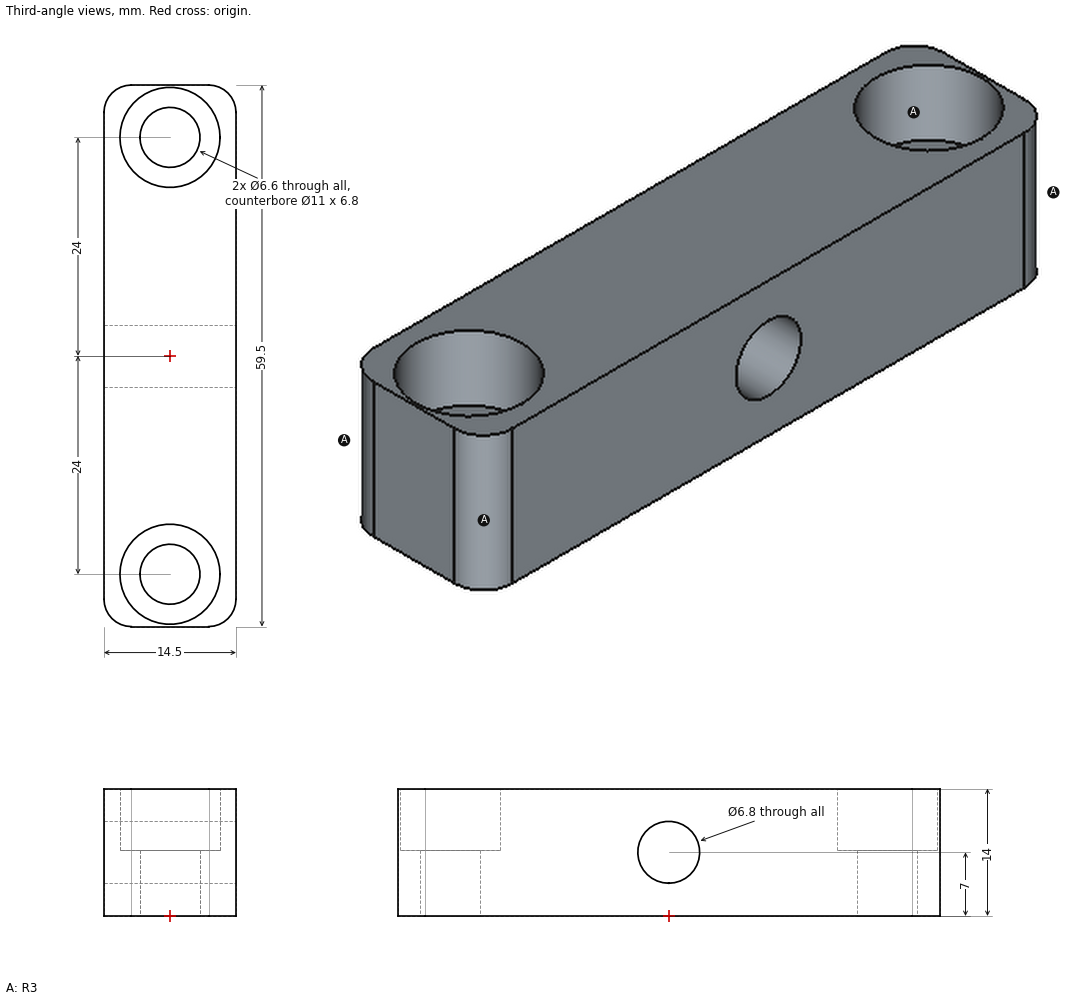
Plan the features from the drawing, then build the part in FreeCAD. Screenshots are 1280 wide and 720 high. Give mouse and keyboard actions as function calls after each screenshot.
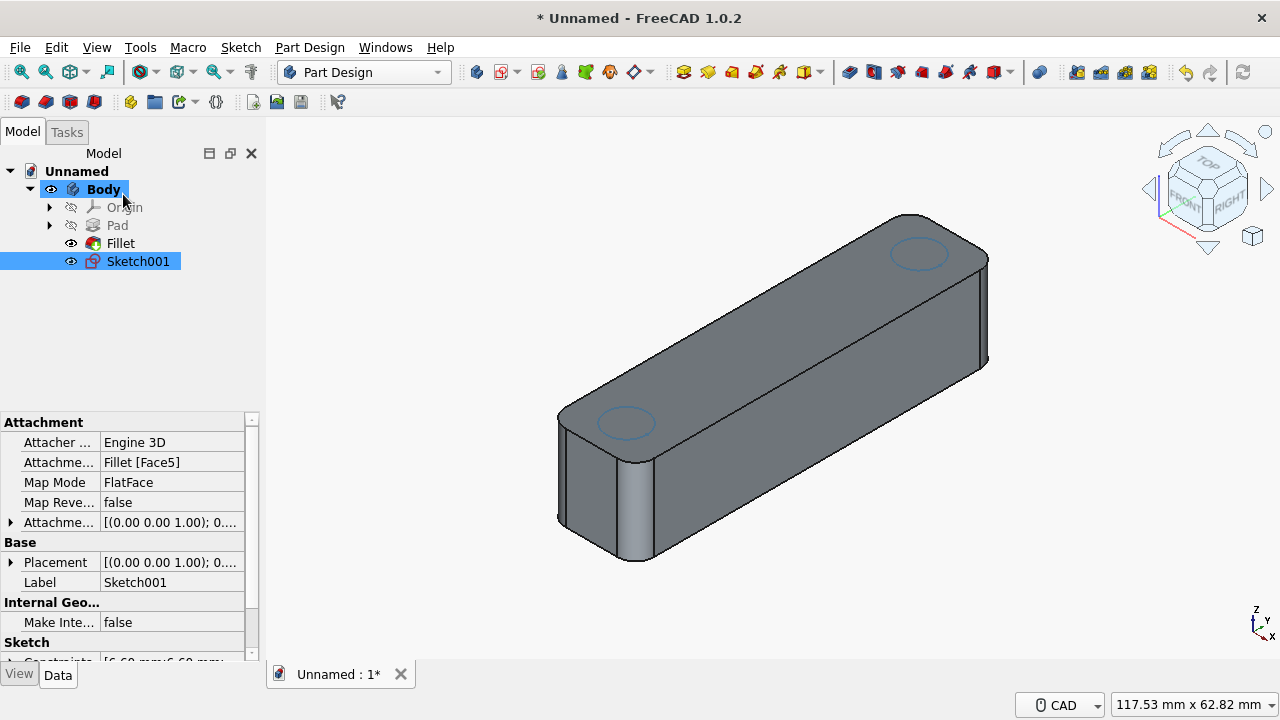
click(874, 72)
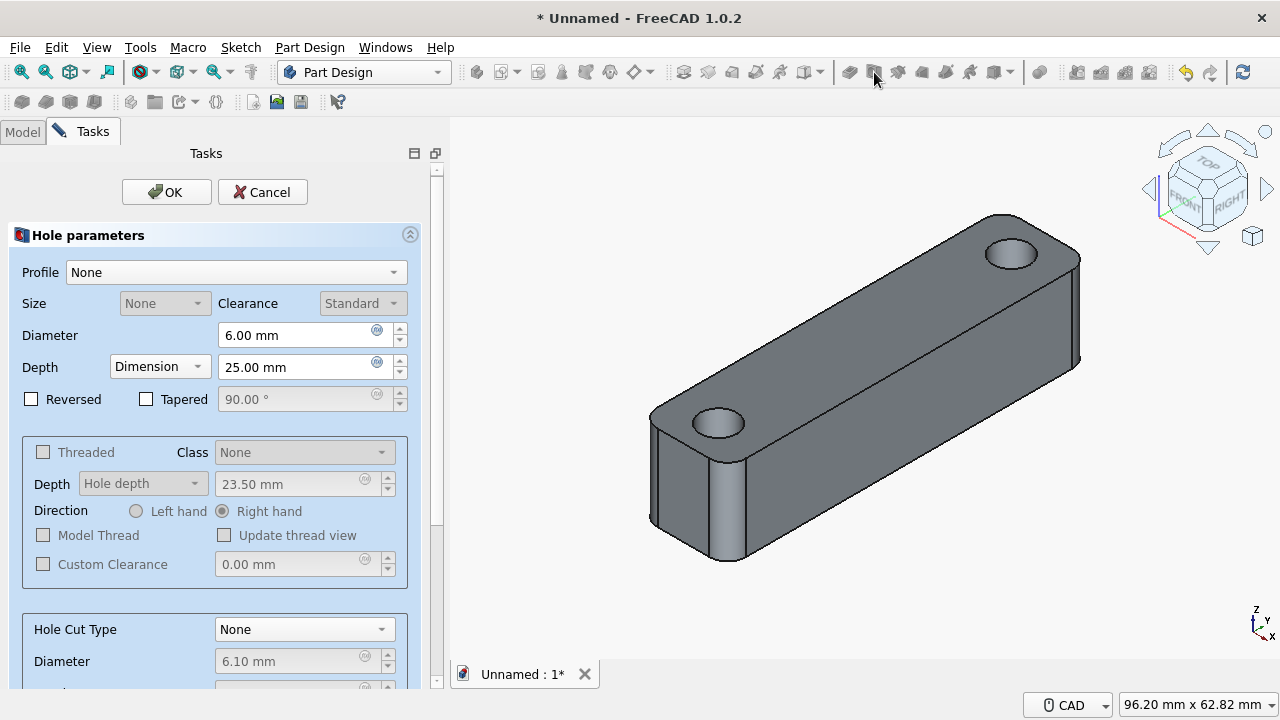
triple_click(305, 335)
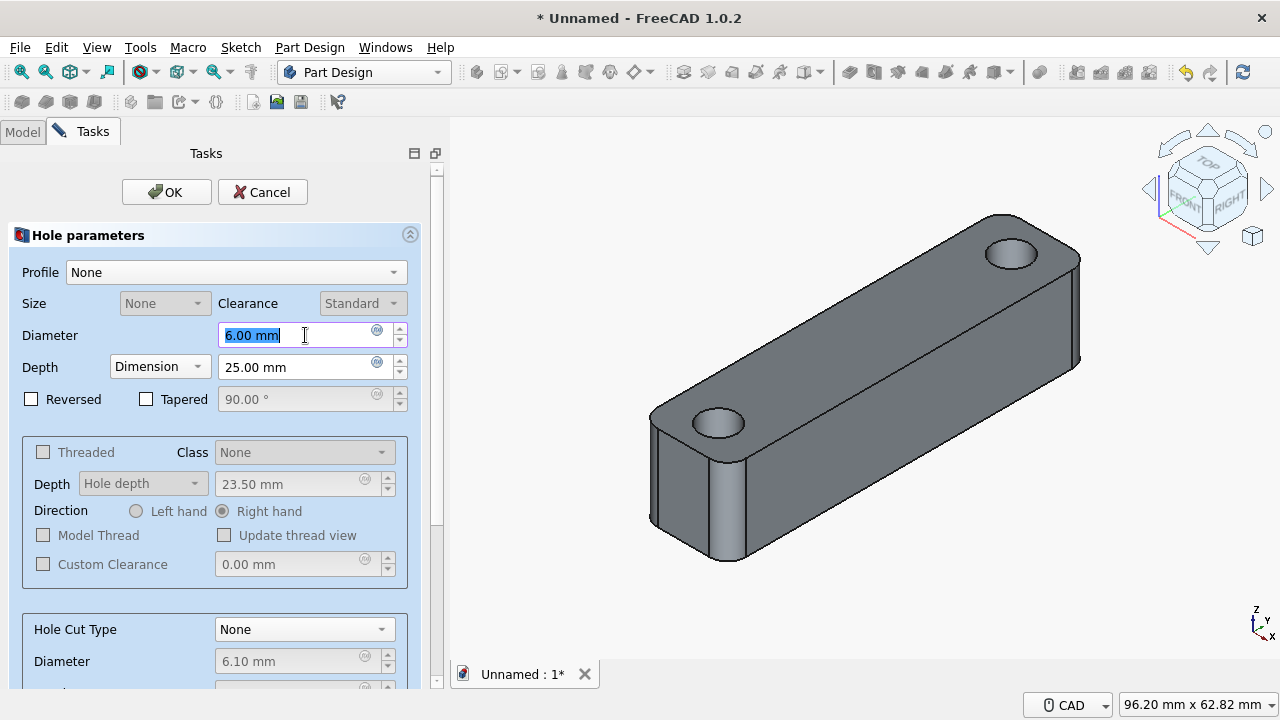
text(6.6)
key(Tab)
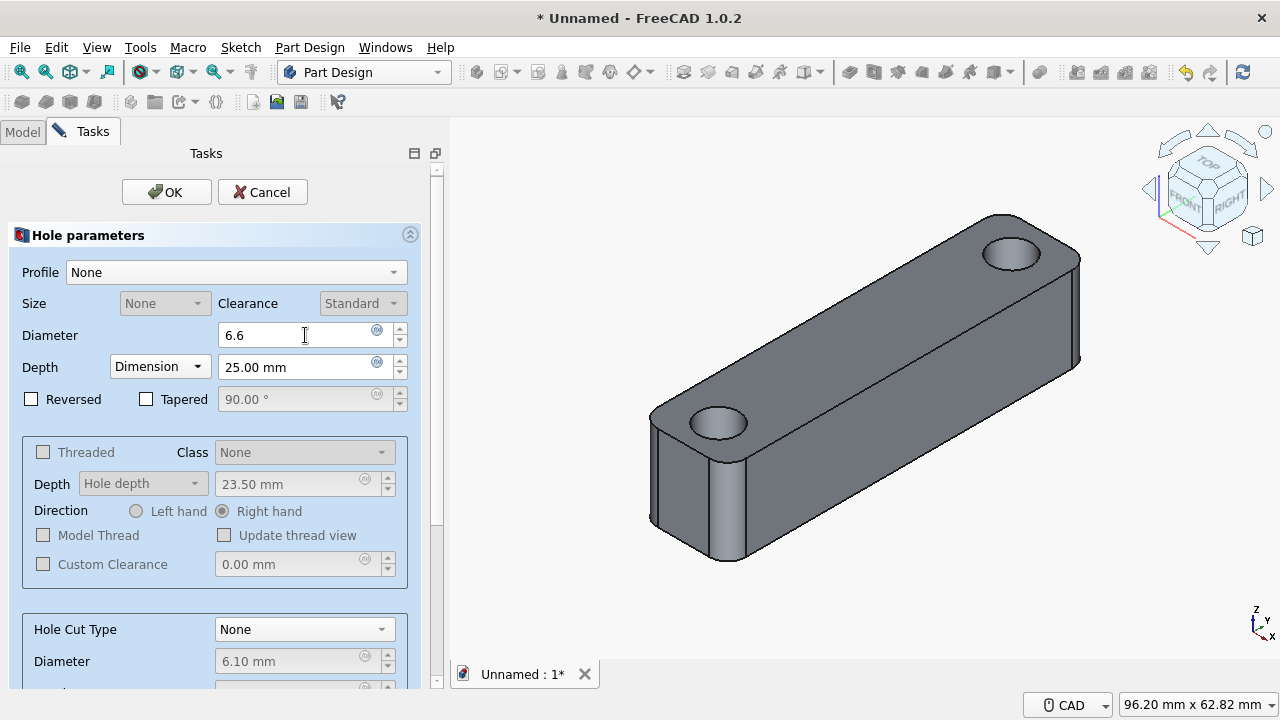
click(161, 366)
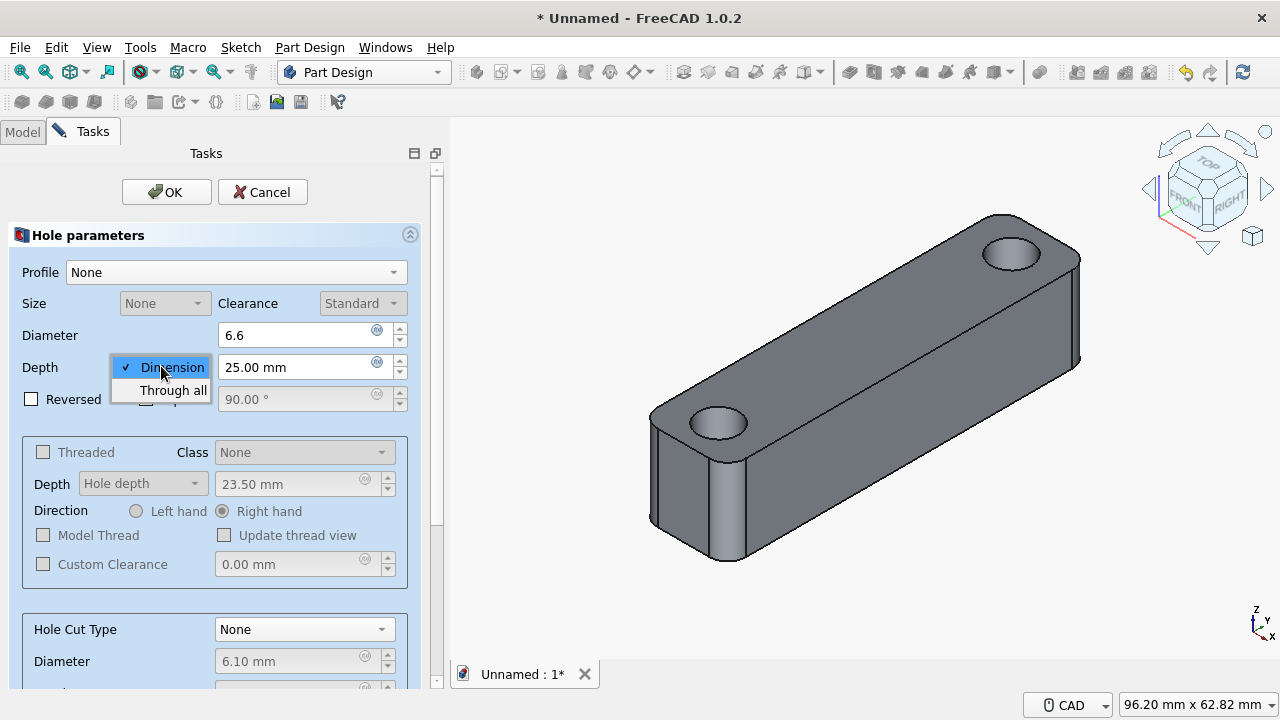
click(160, 390)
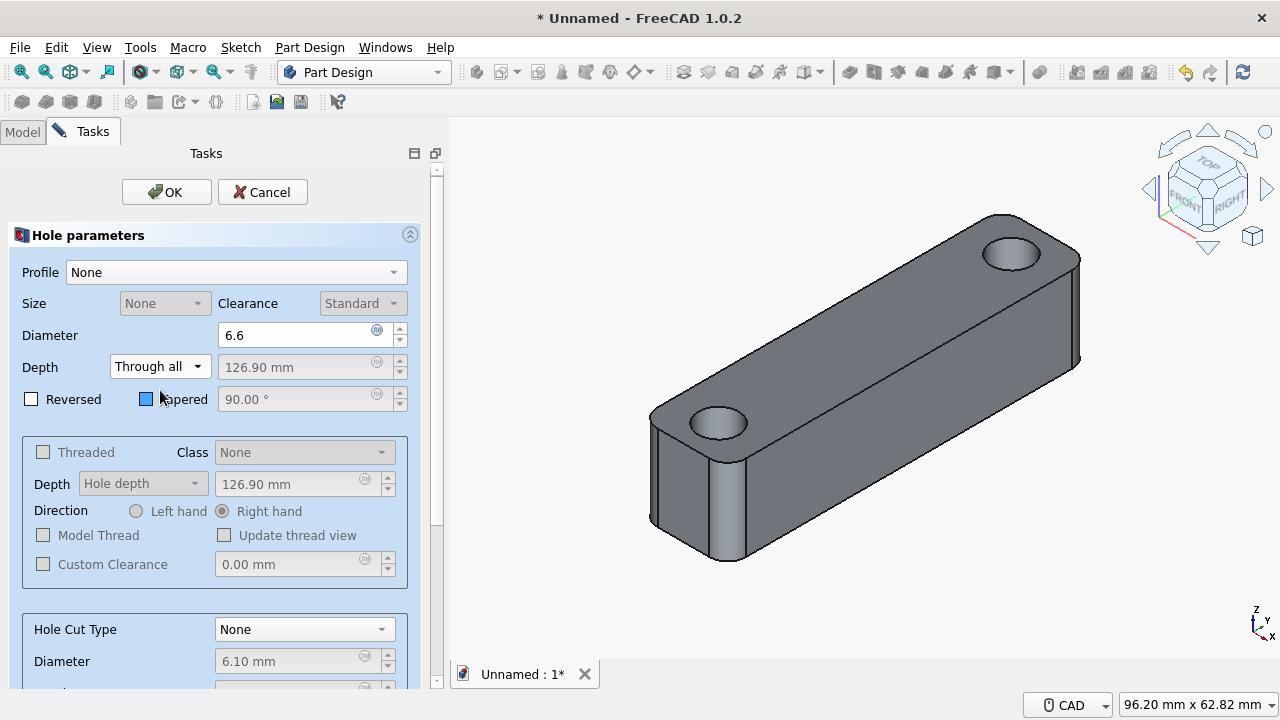
click(306, 630)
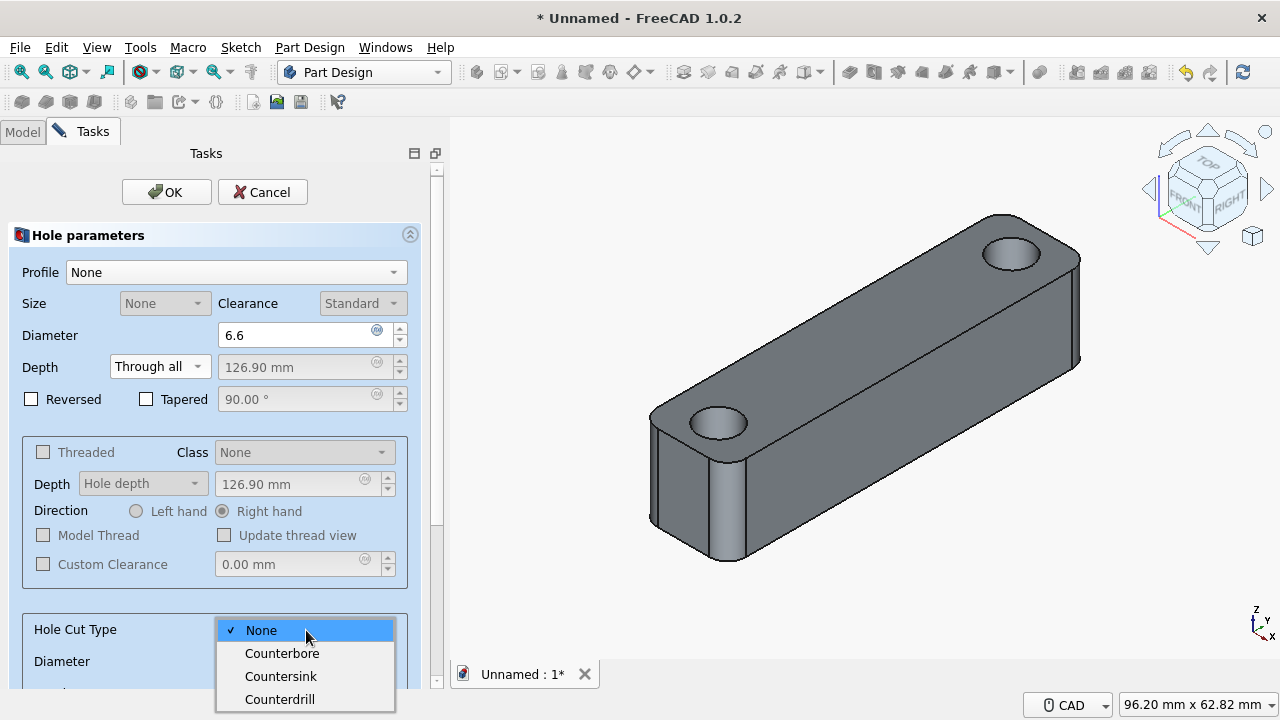
click(304, 654)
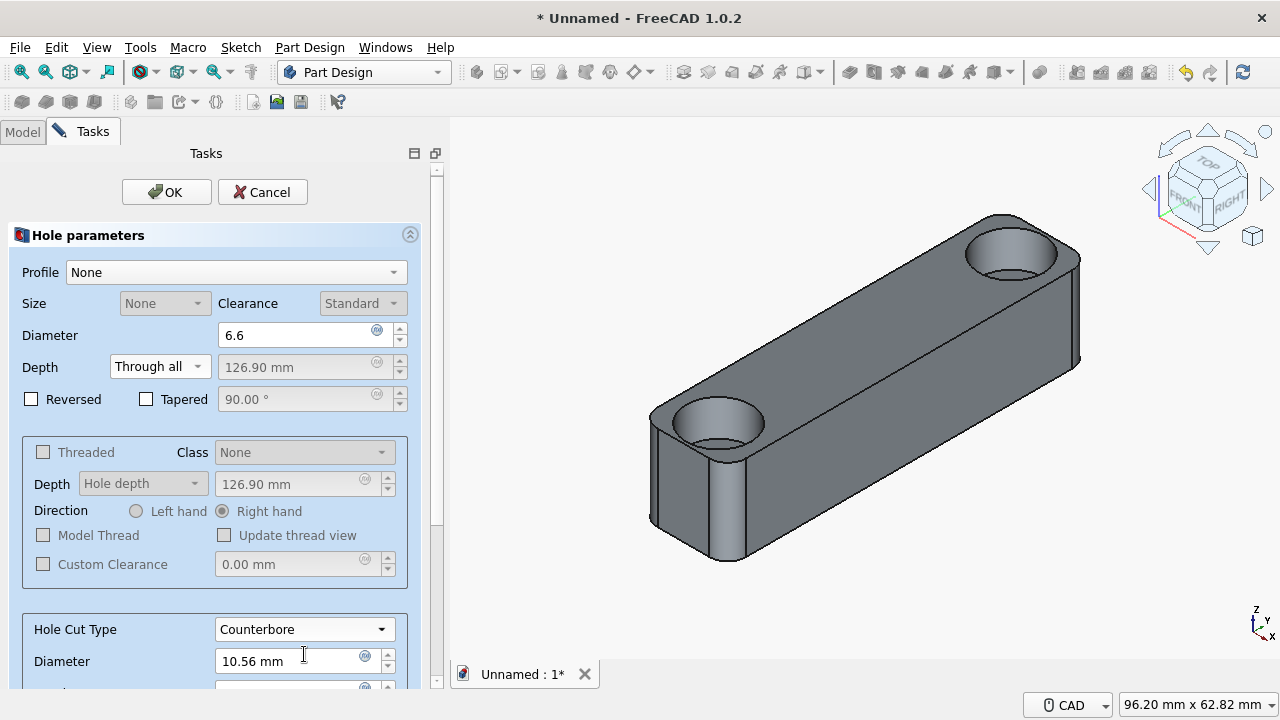
triple_click(298, 661)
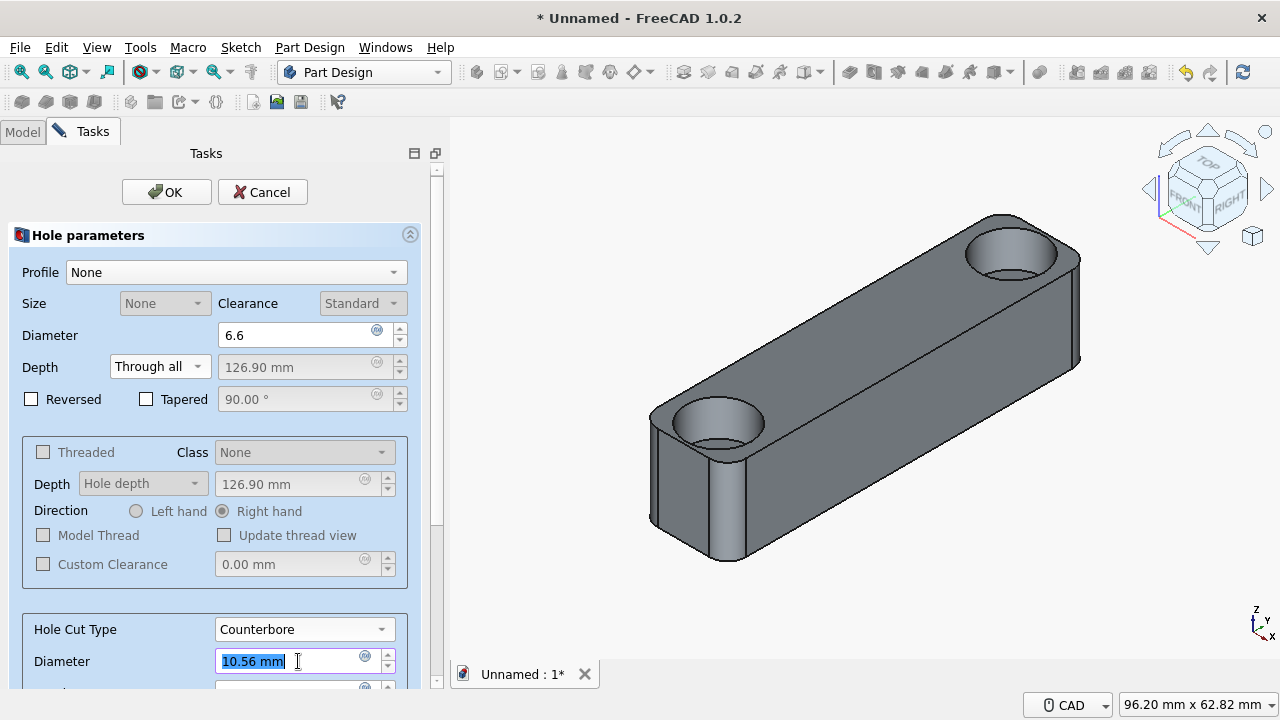
text(11)
key(Tab)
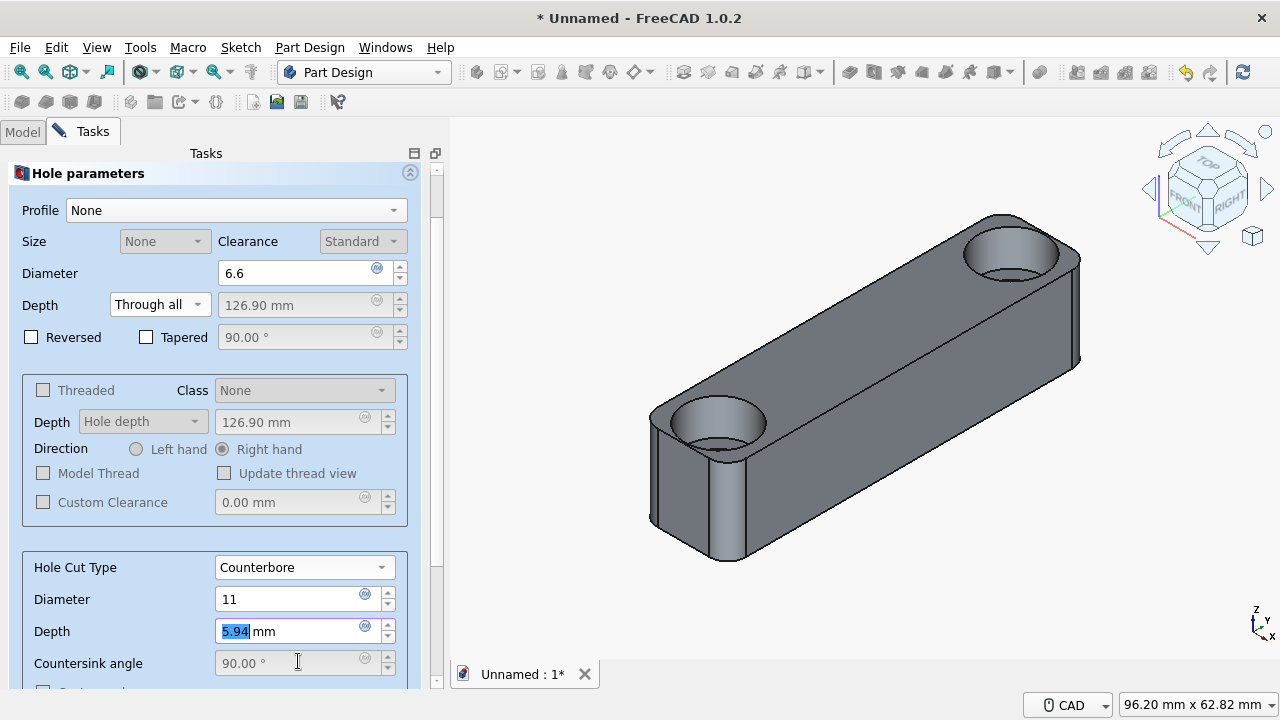
text(6.8)
key(Tab)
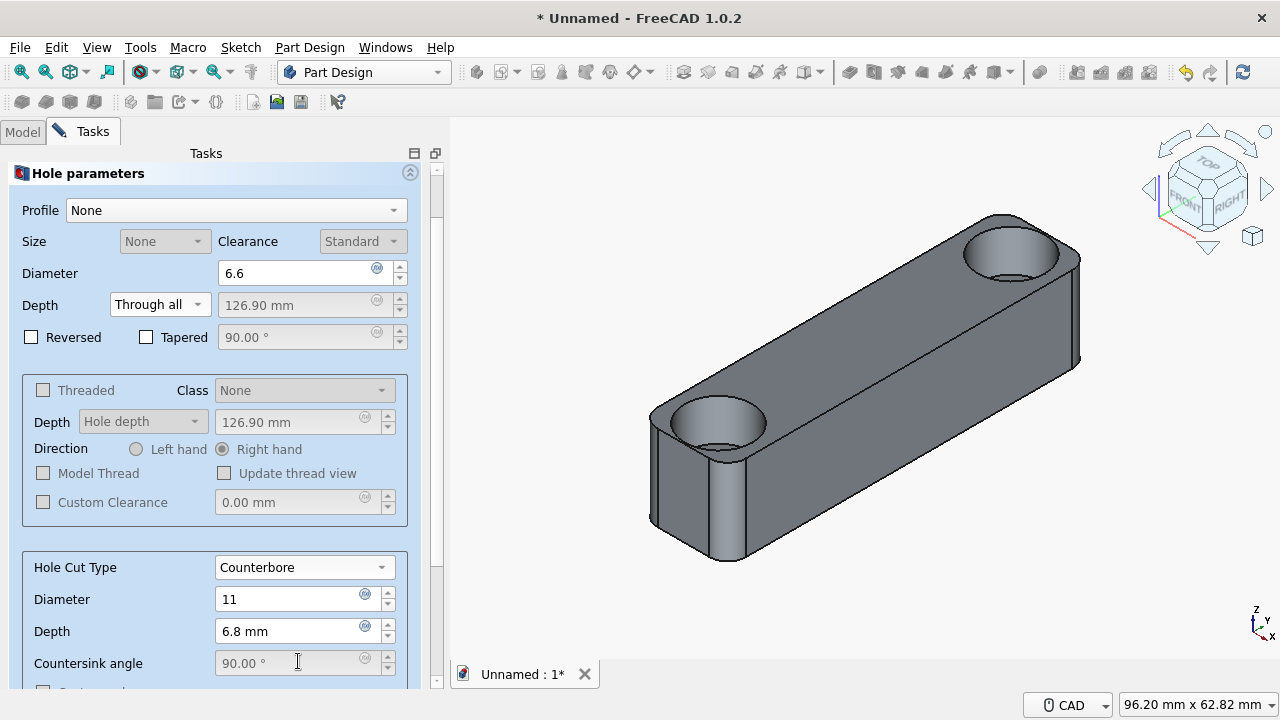
scroll(437, 426, up, 2)